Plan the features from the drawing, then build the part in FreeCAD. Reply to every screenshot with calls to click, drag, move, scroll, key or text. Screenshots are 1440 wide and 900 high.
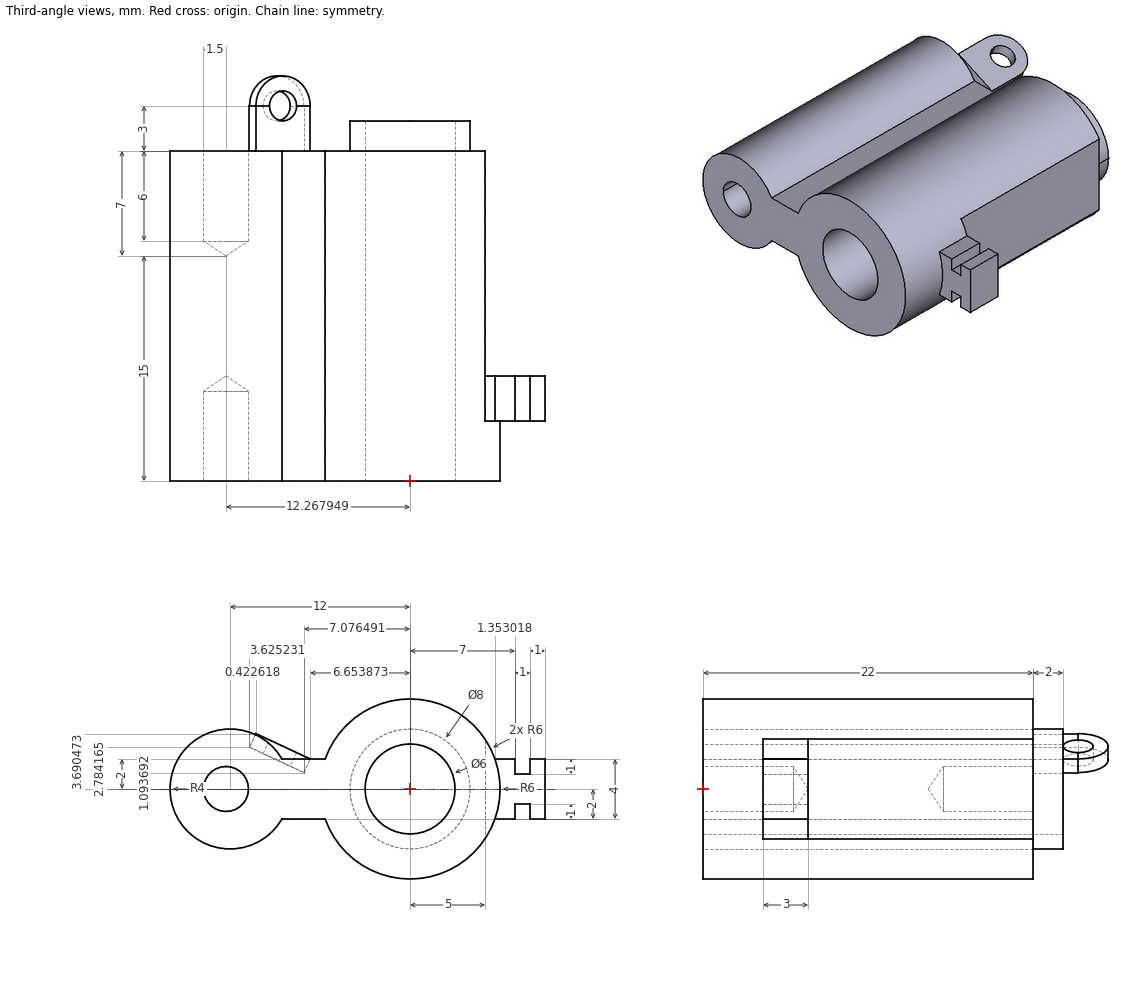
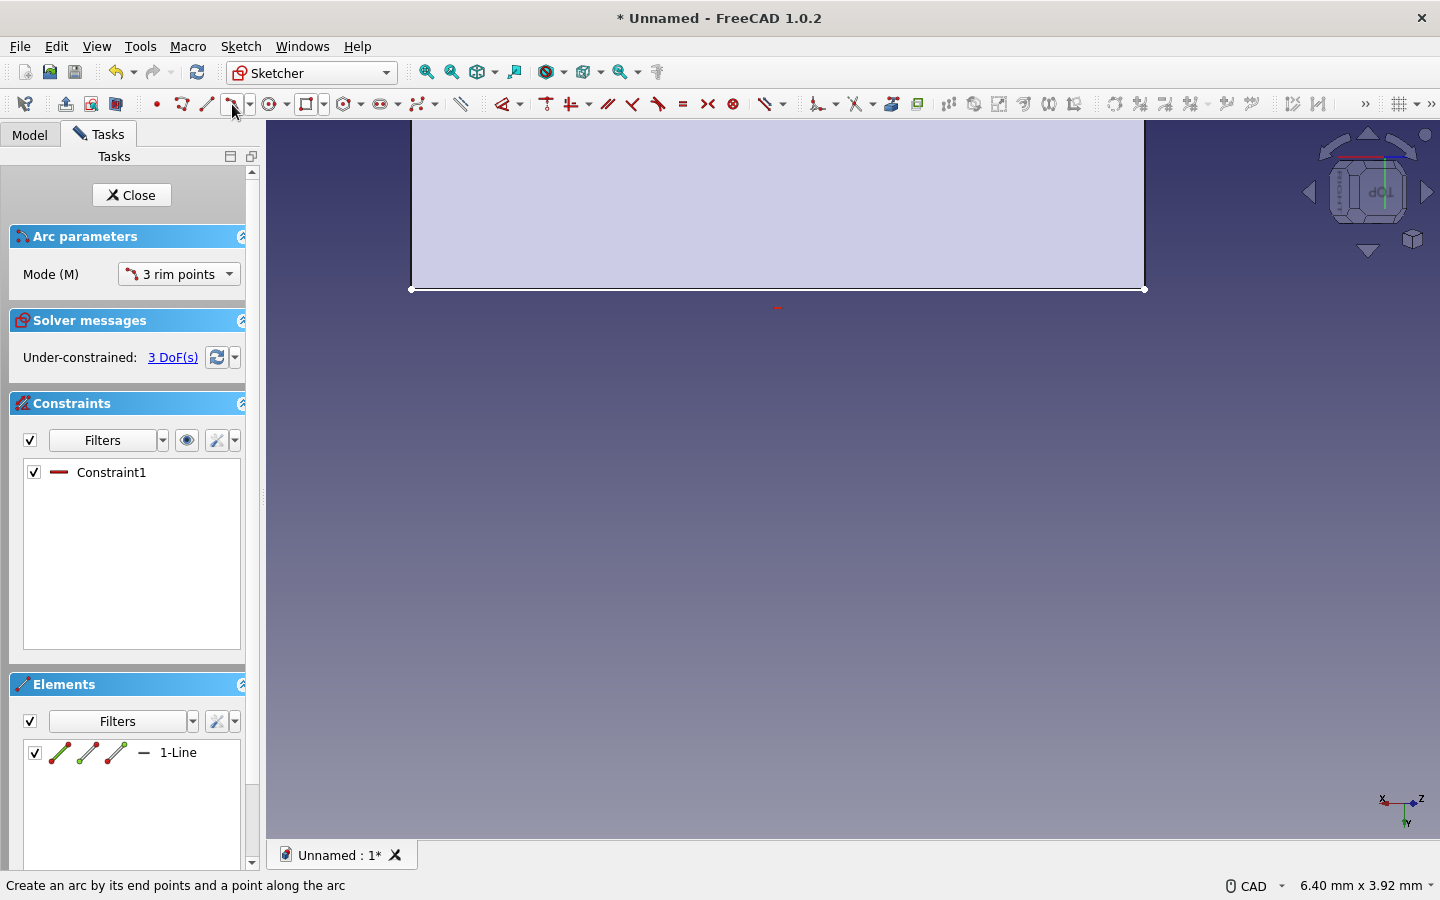
click(411, 290)
click(1145, 290)
click(778, 656)
key(Escape)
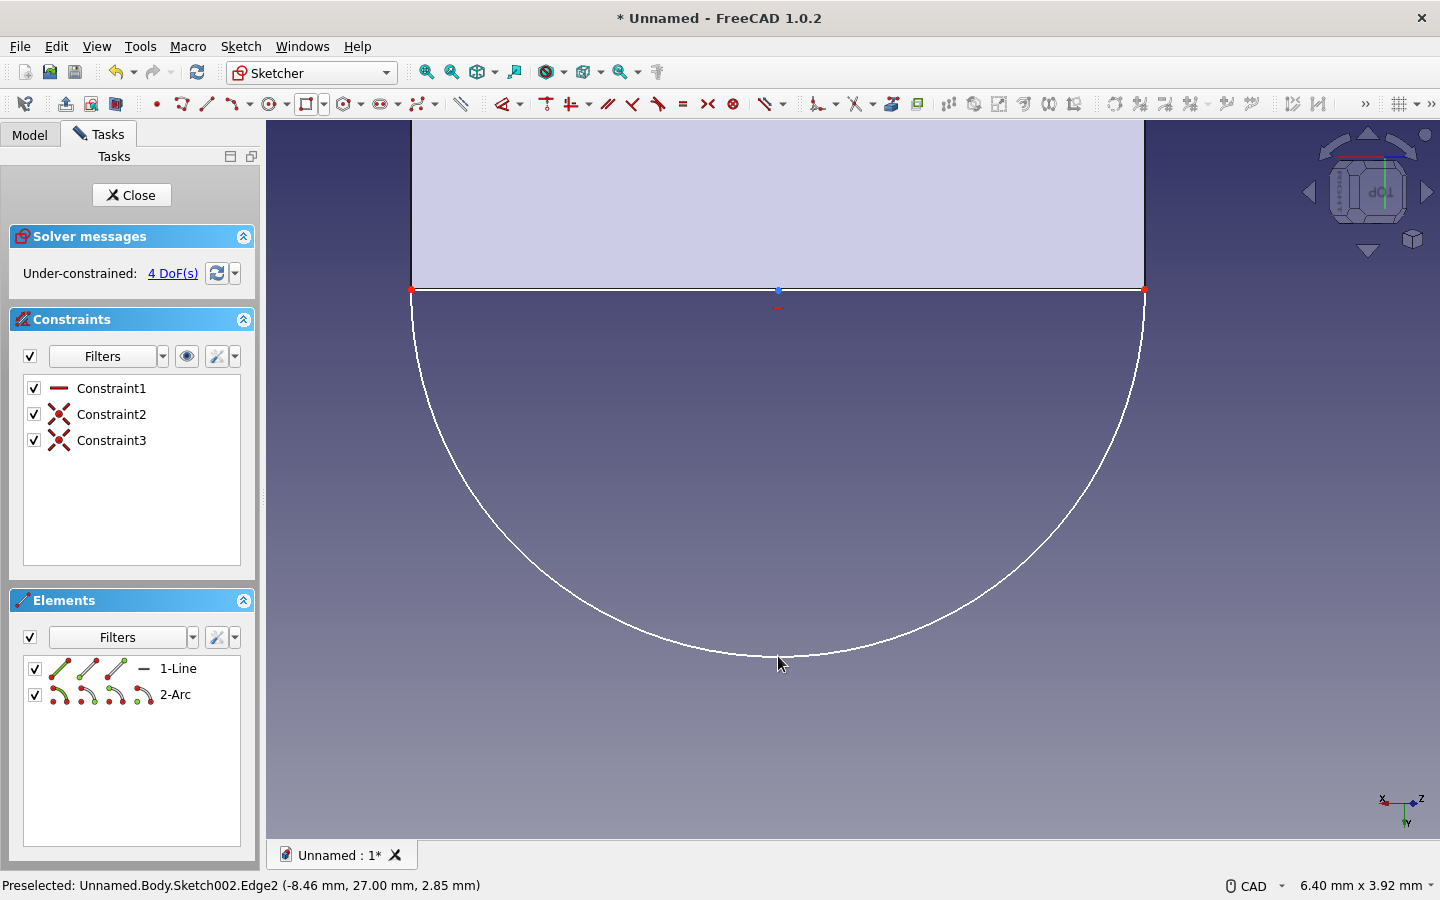
click(502, 104)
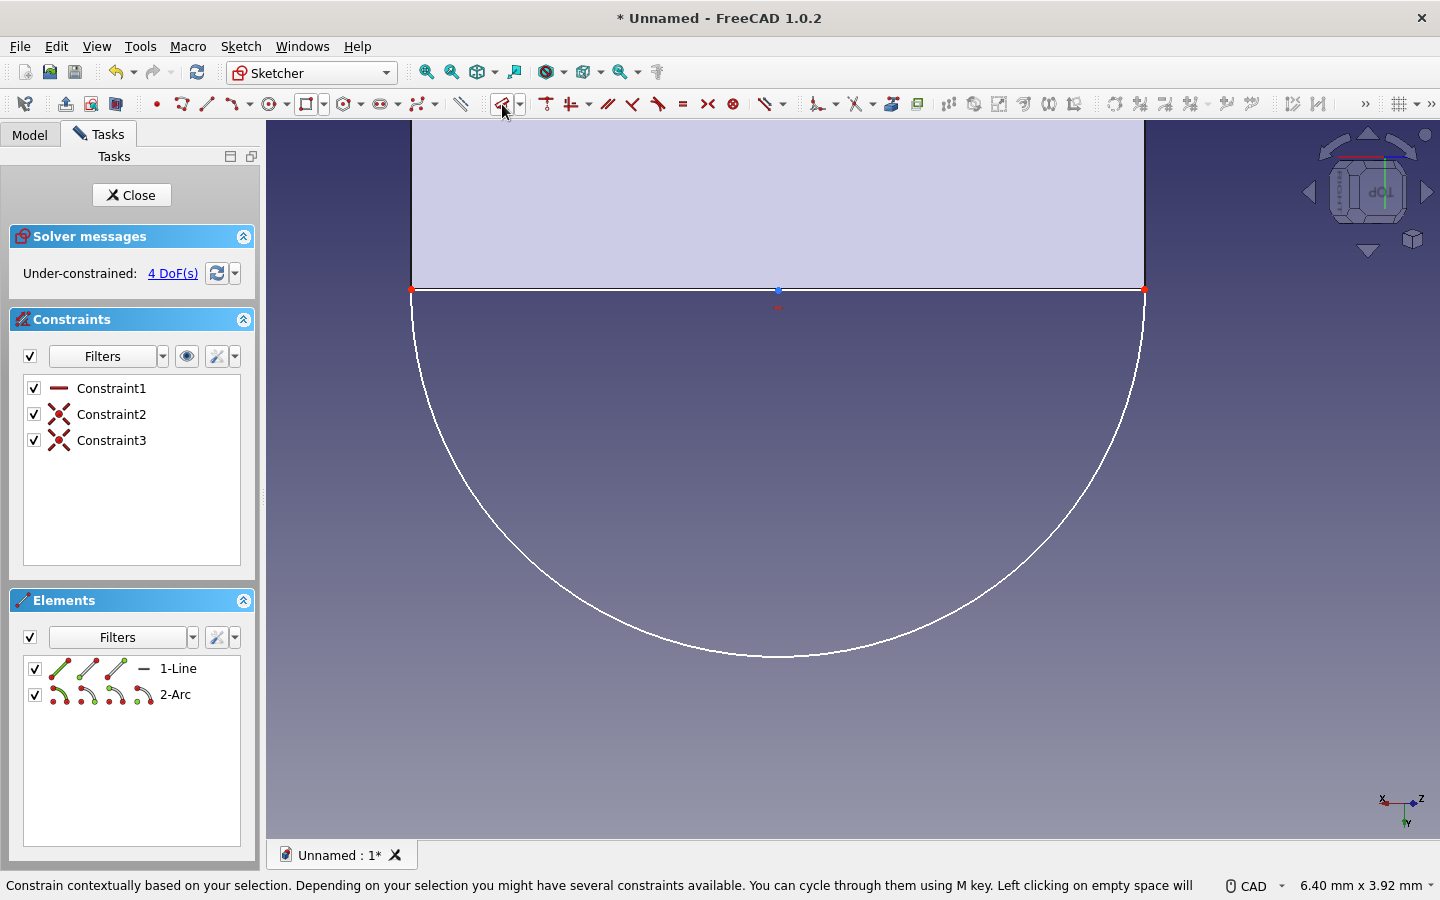
click(562, 587)
click(543, 613)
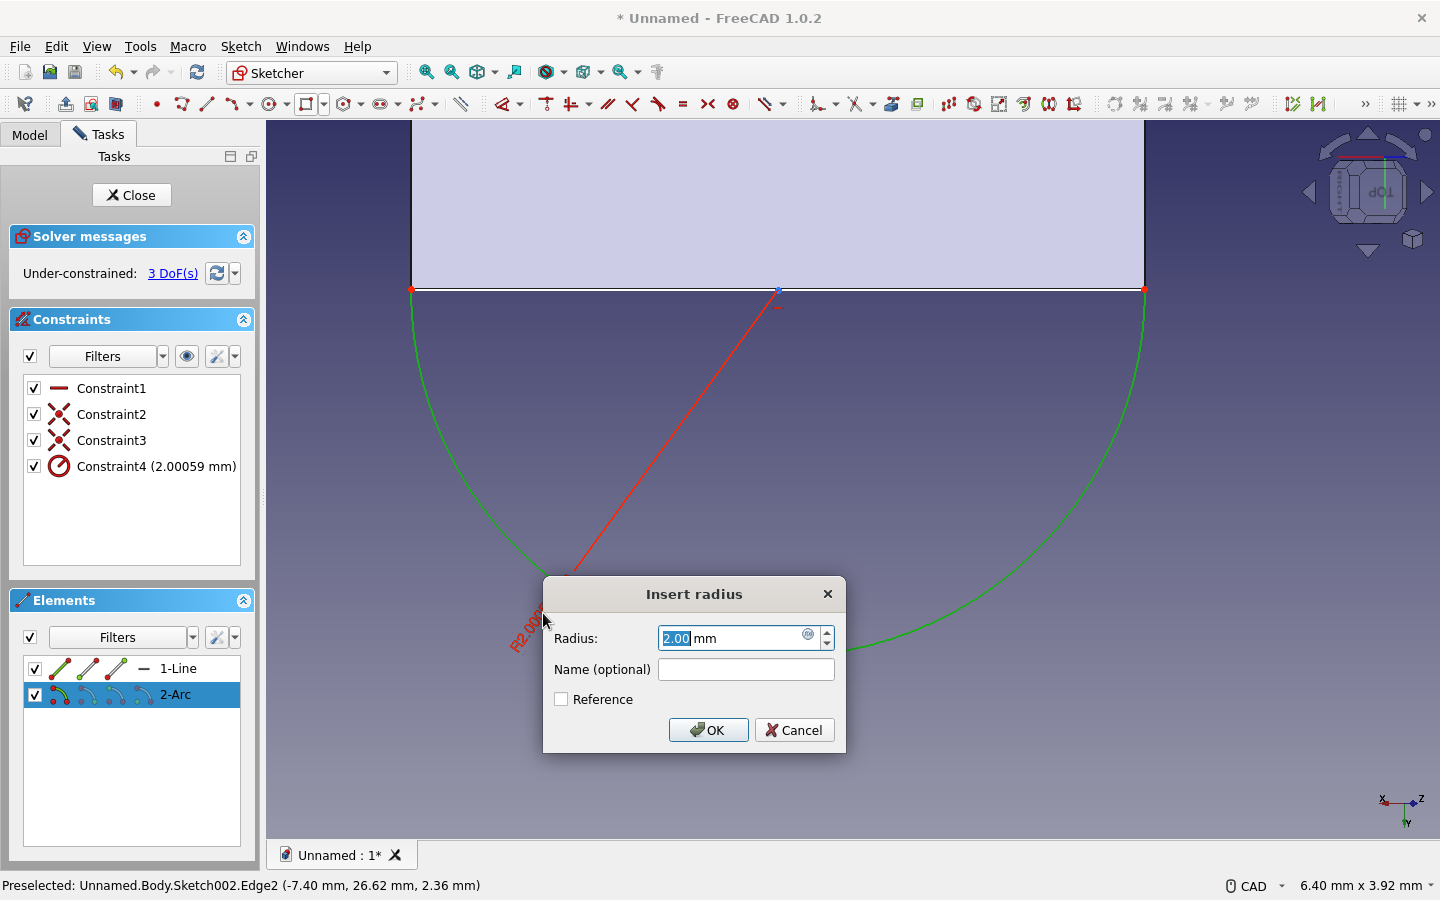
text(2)
key(Return)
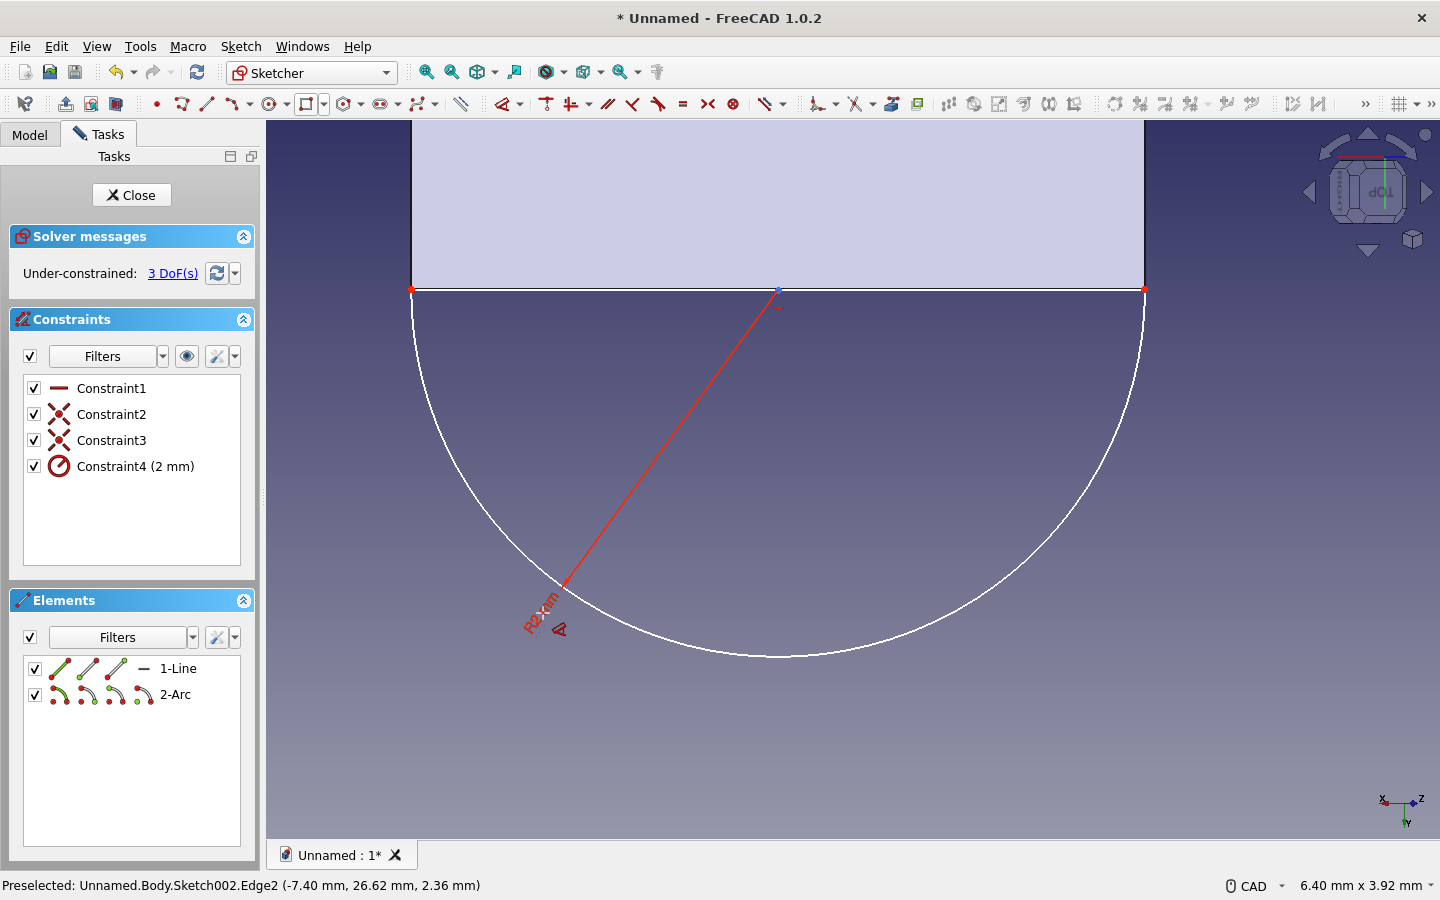
click(1145, 290)
click(1179, 219)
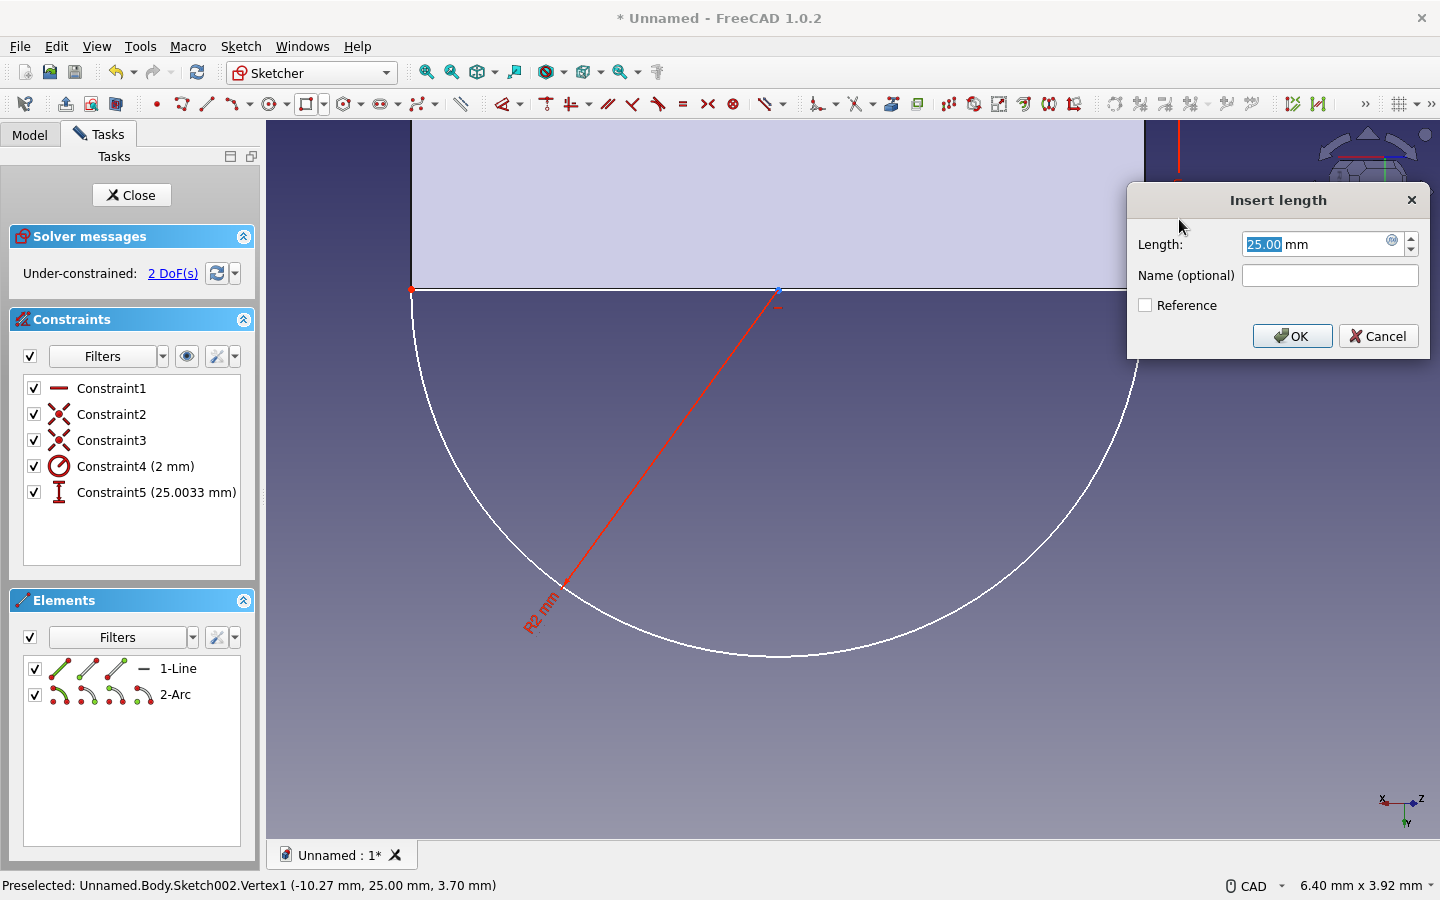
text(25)
key(Return)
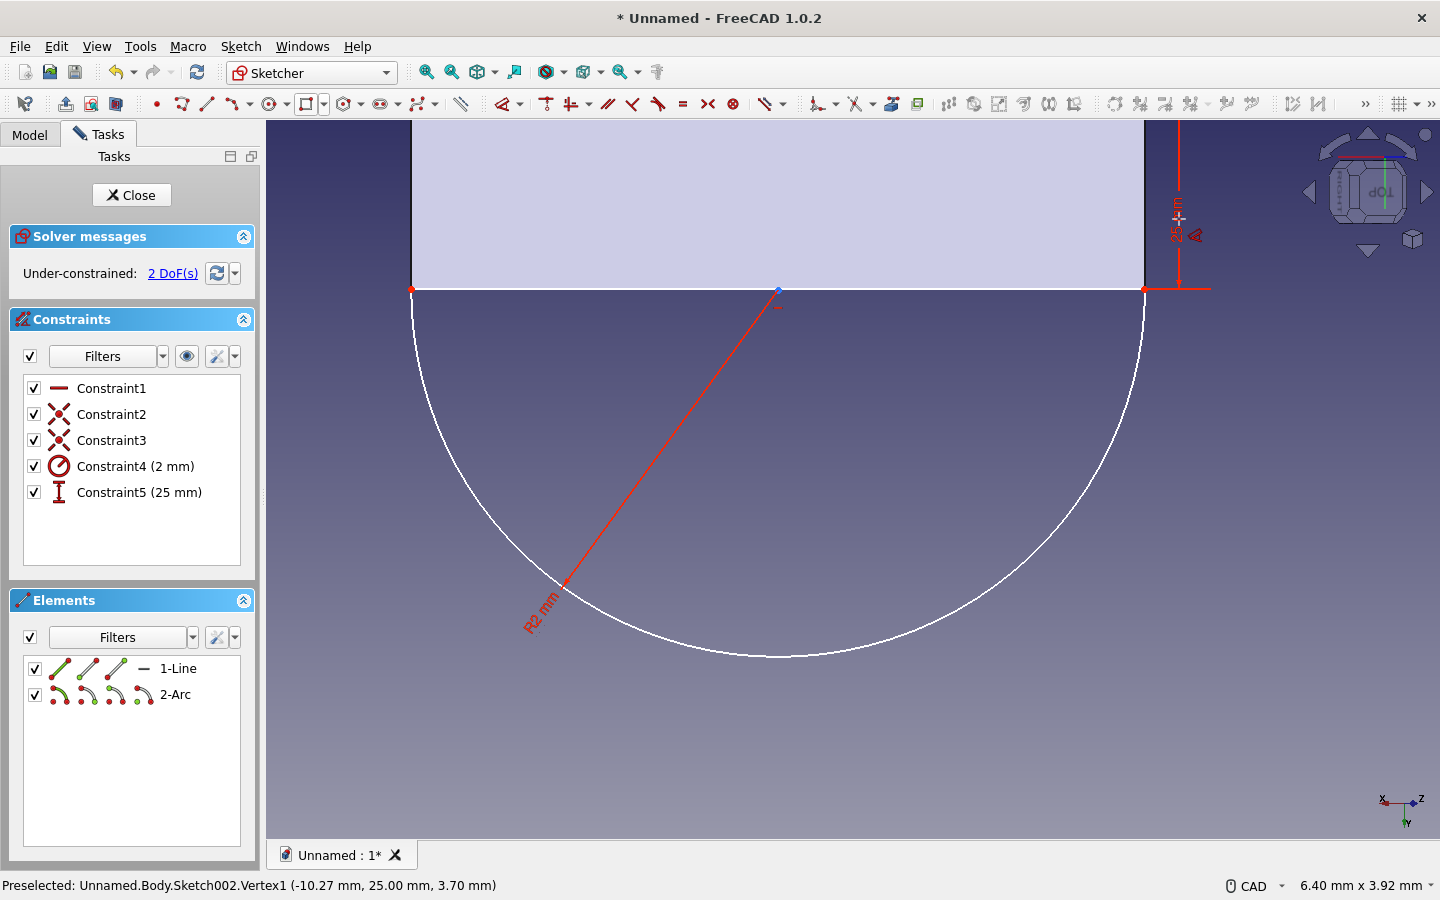
click(778, 290)
click(812, 219)